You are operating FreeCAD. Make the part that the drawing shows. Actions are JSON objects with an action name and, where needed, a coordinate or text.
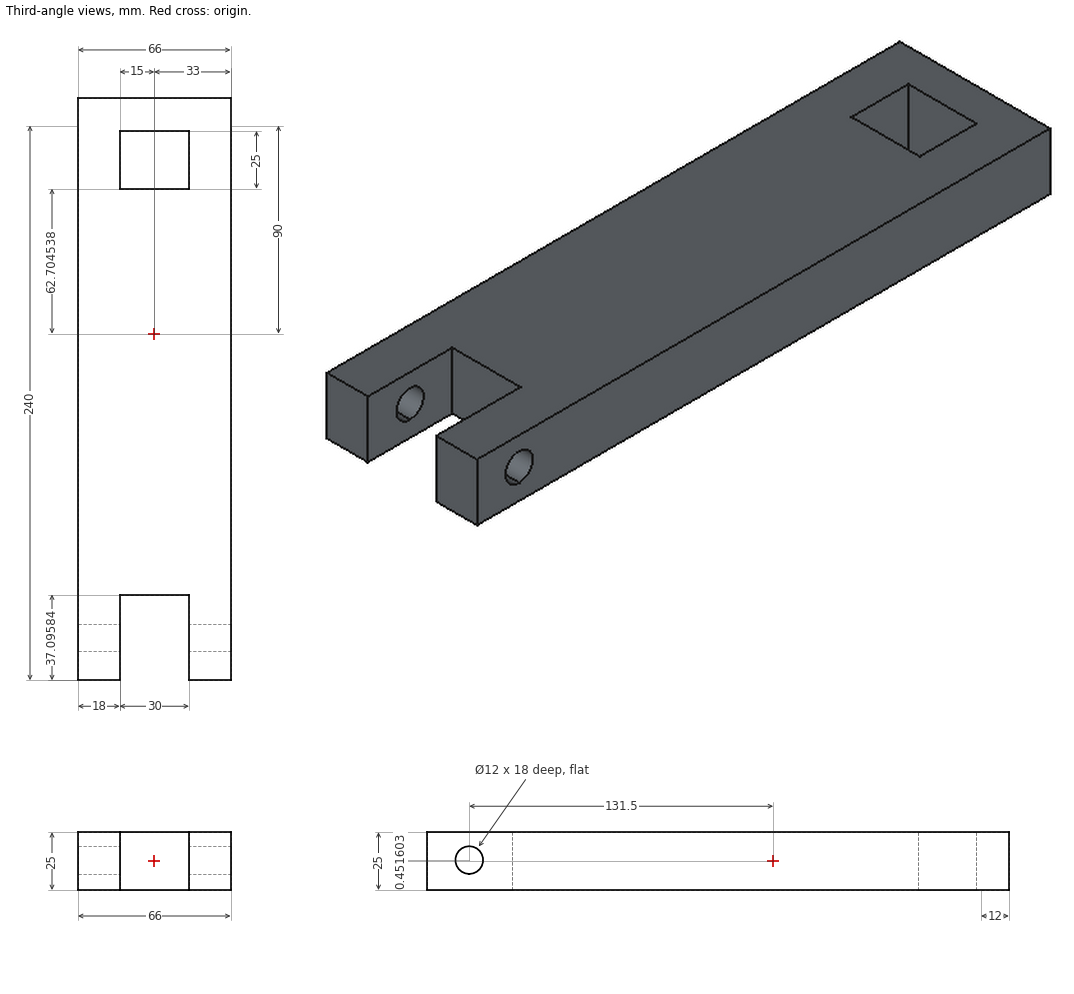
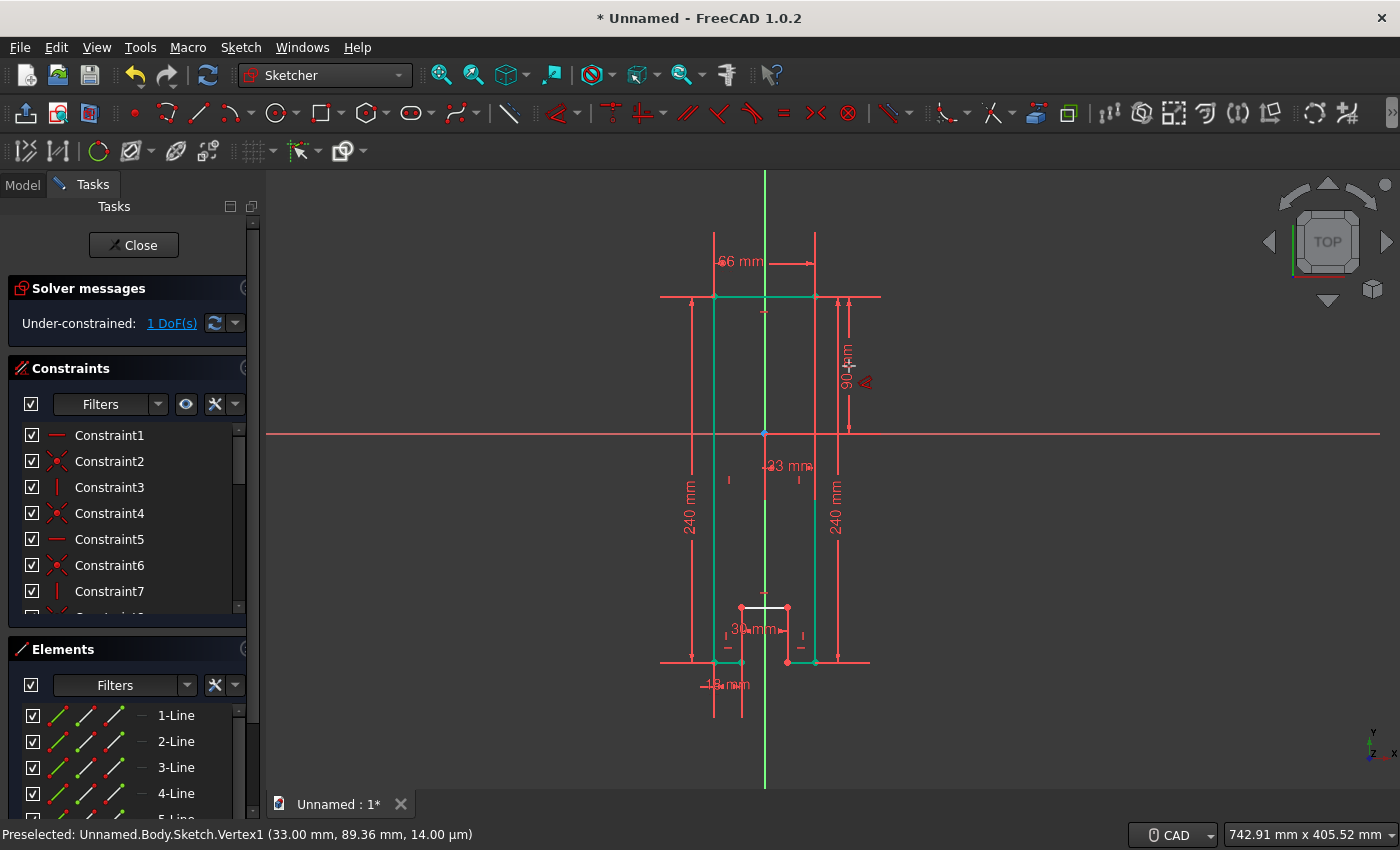
{"action": "left_click", "coordinate": [742, 646]}
{"action": "left_click", "coordinate": [684, 635]}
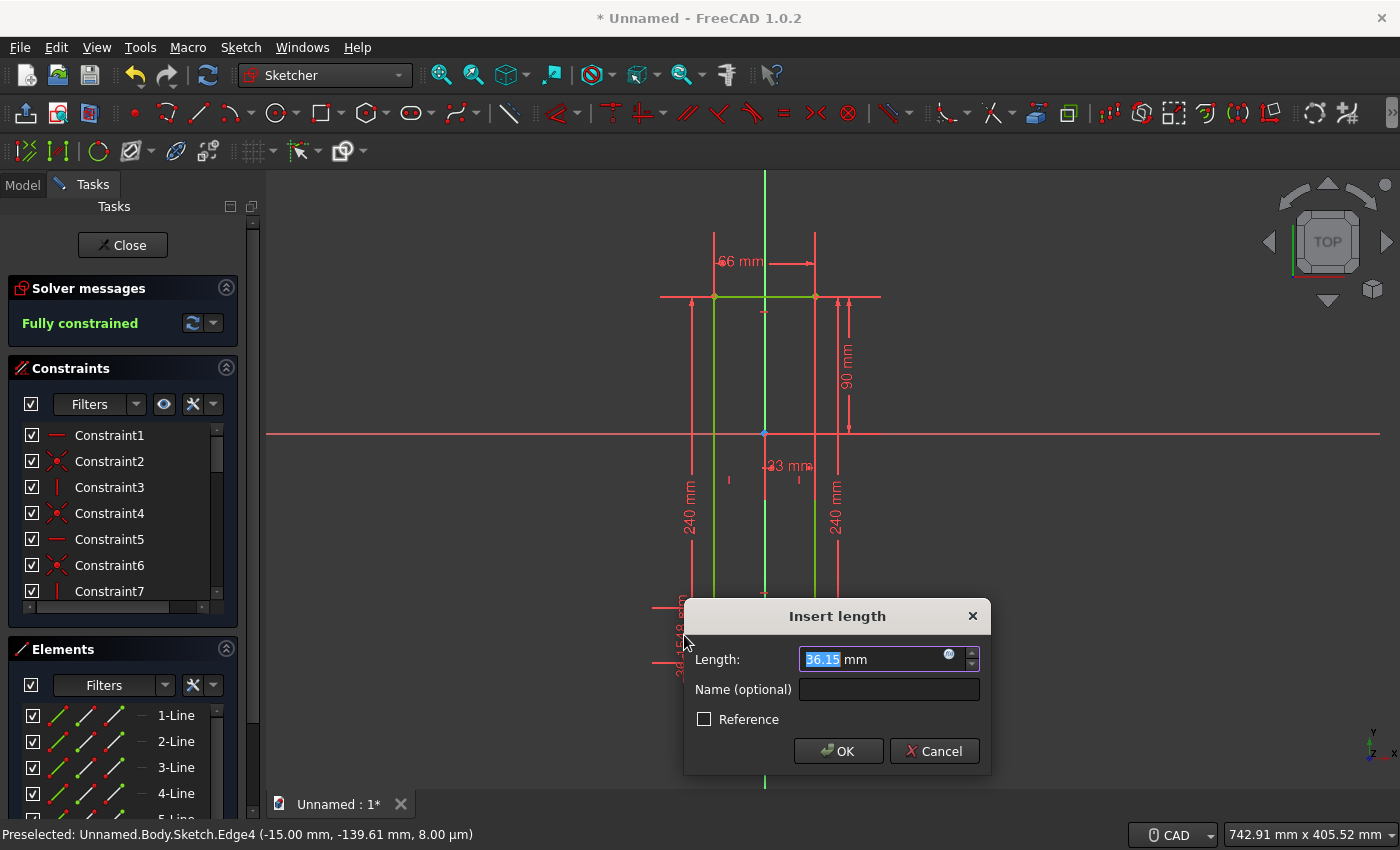
{"action": "type", "text": "37.09584"}
{"action": "key", "text": "Return"}
{"action": "key", "text": "Escape"}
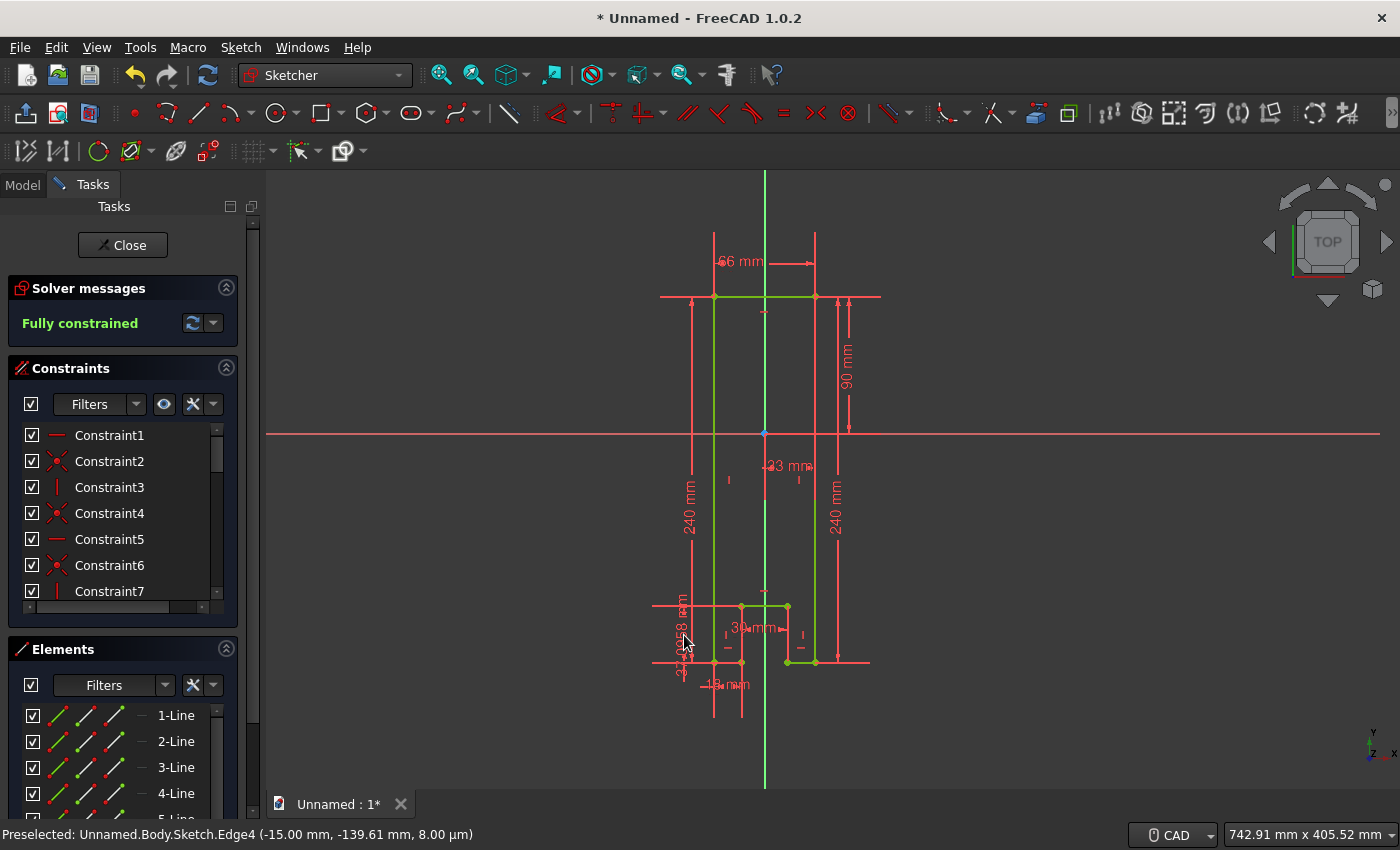
{"action": "left_click", "coordinate": [123, 245]}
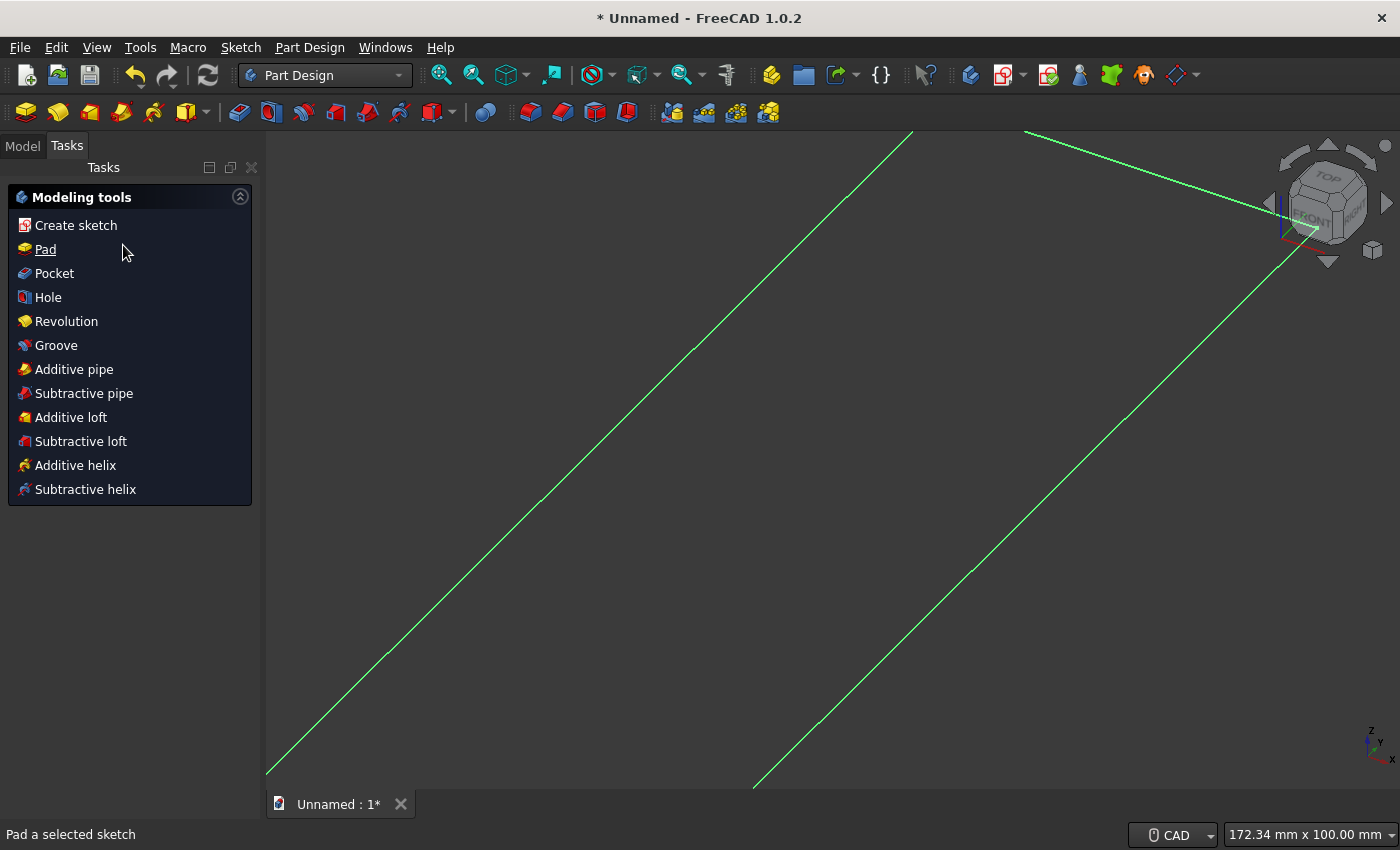
{"action": "left_click", "coordinate": [26, 112]}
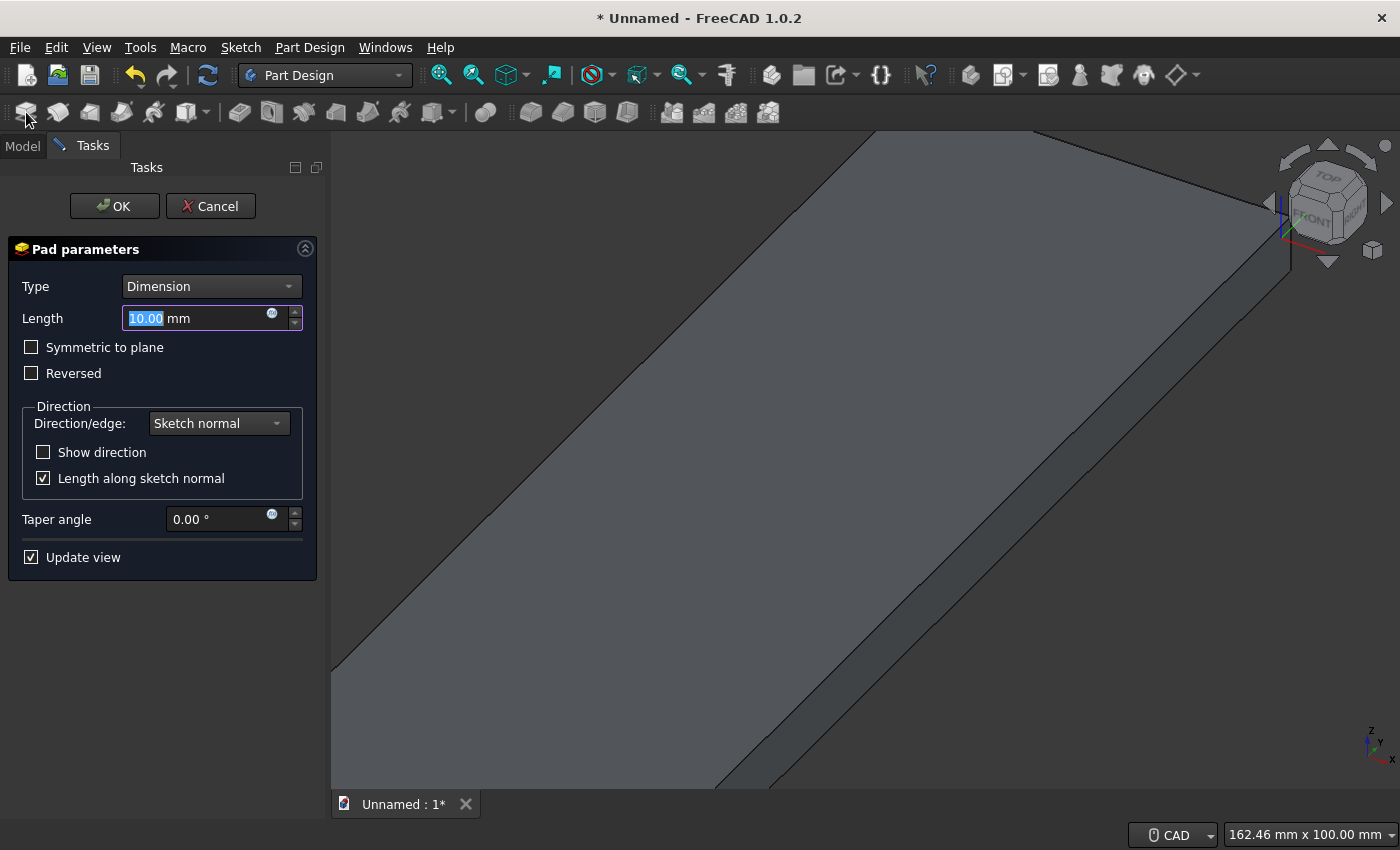
{"action": "type", "text": "25"}
{"action": "key", "text": "Tab"}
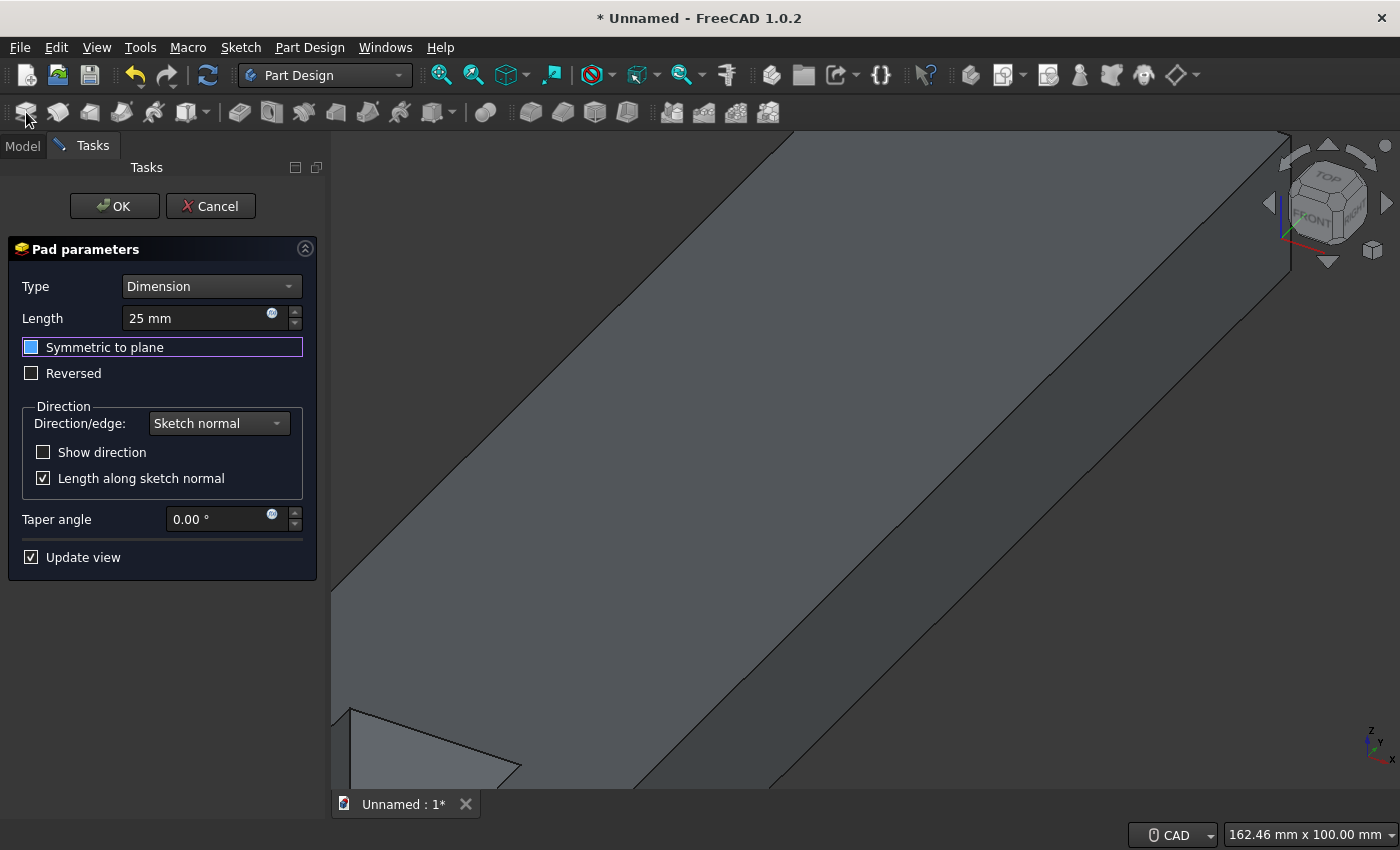
{"action": "left_click", "coordinate": [30, 347]}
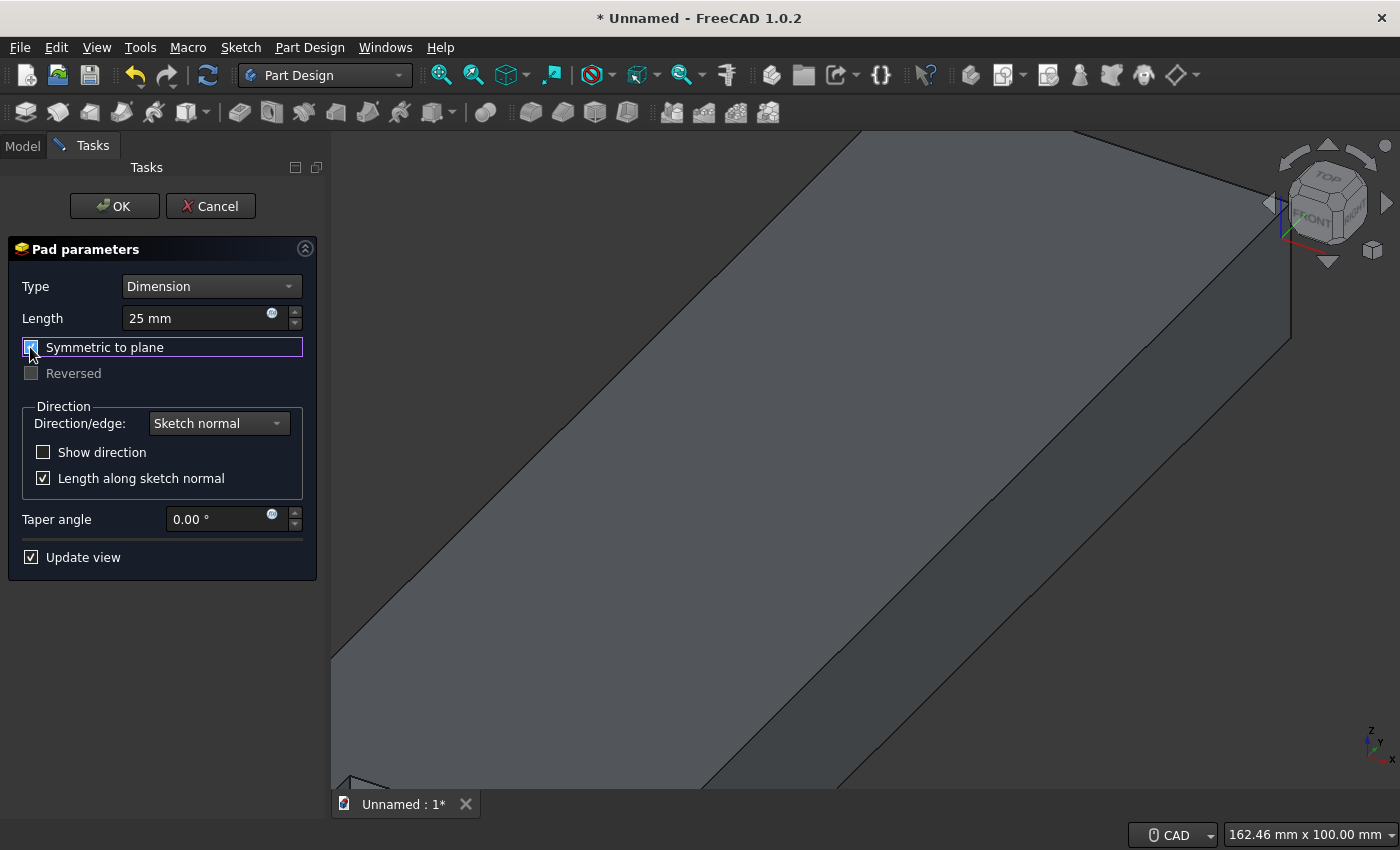
{"action": "left_click", "coordinate": [115, 206]}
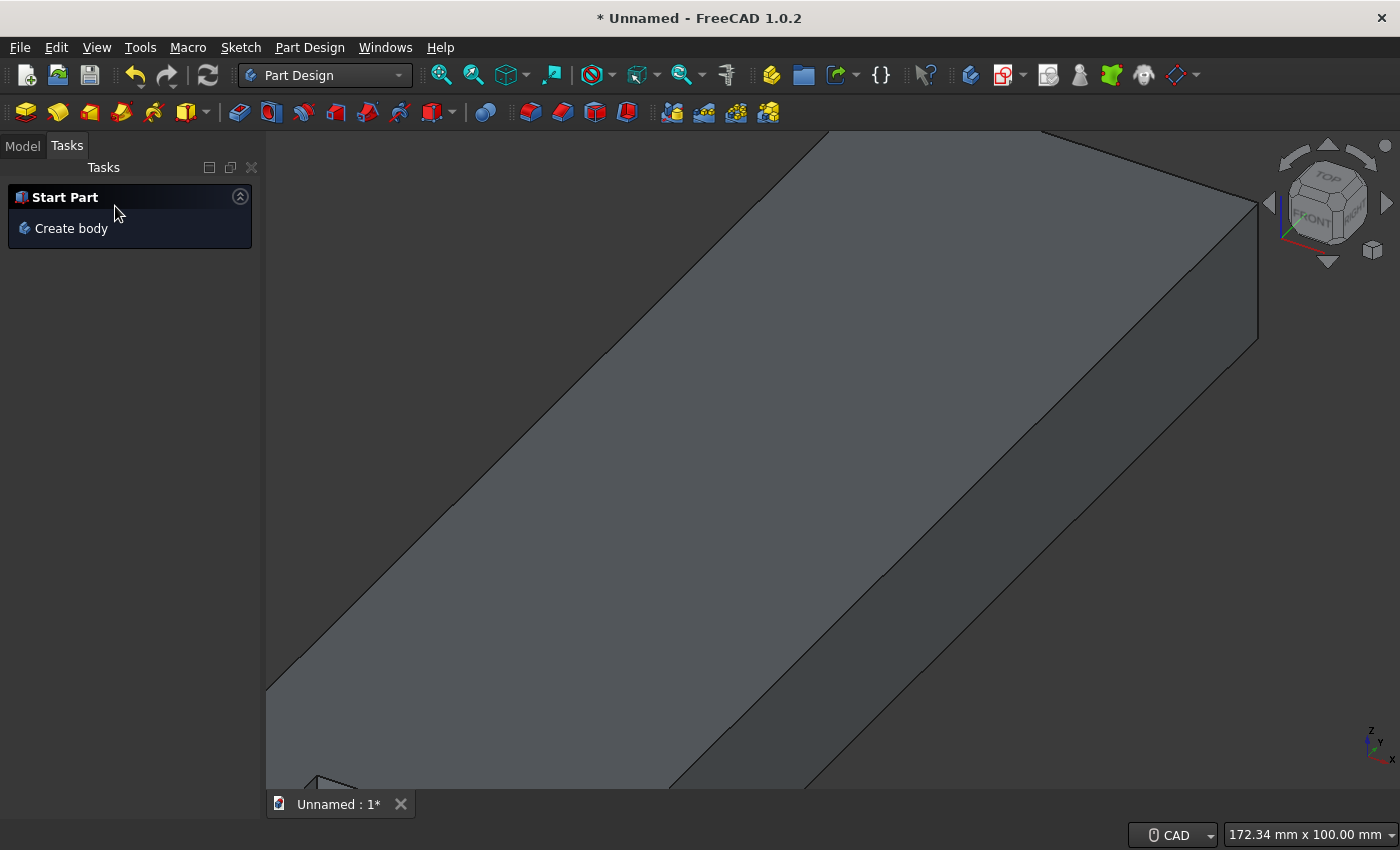
{"action": "left_click", "coordinate": [442, 76]}